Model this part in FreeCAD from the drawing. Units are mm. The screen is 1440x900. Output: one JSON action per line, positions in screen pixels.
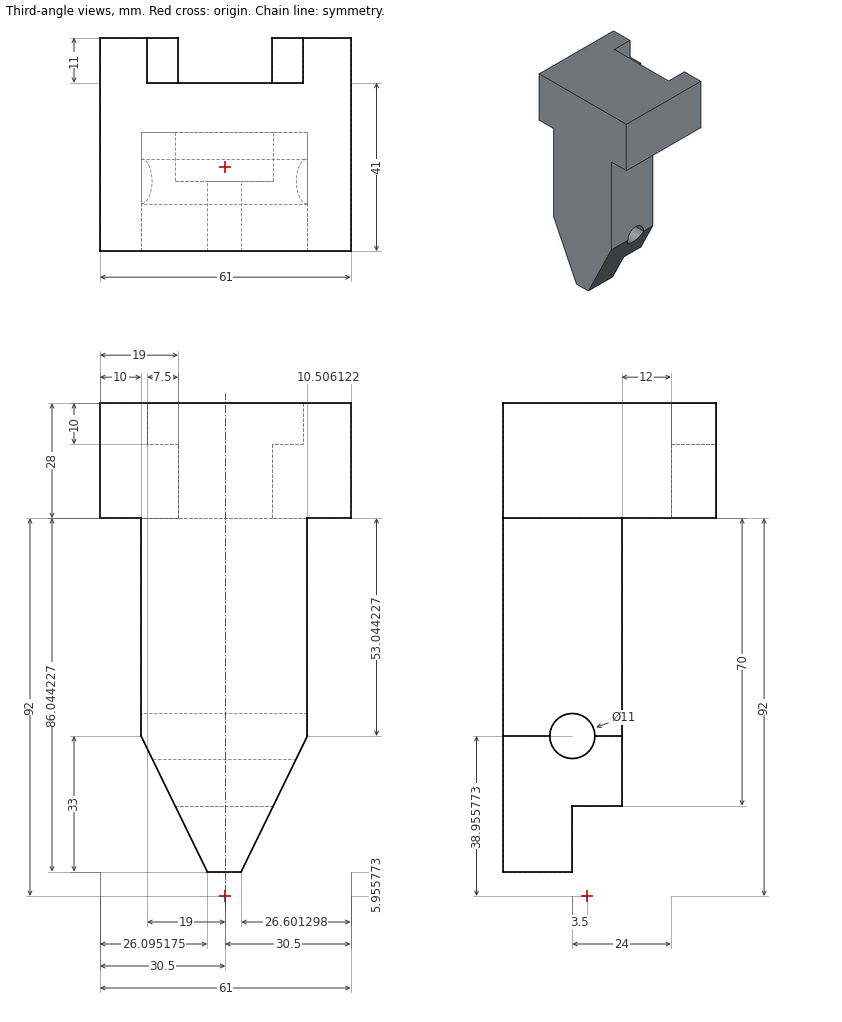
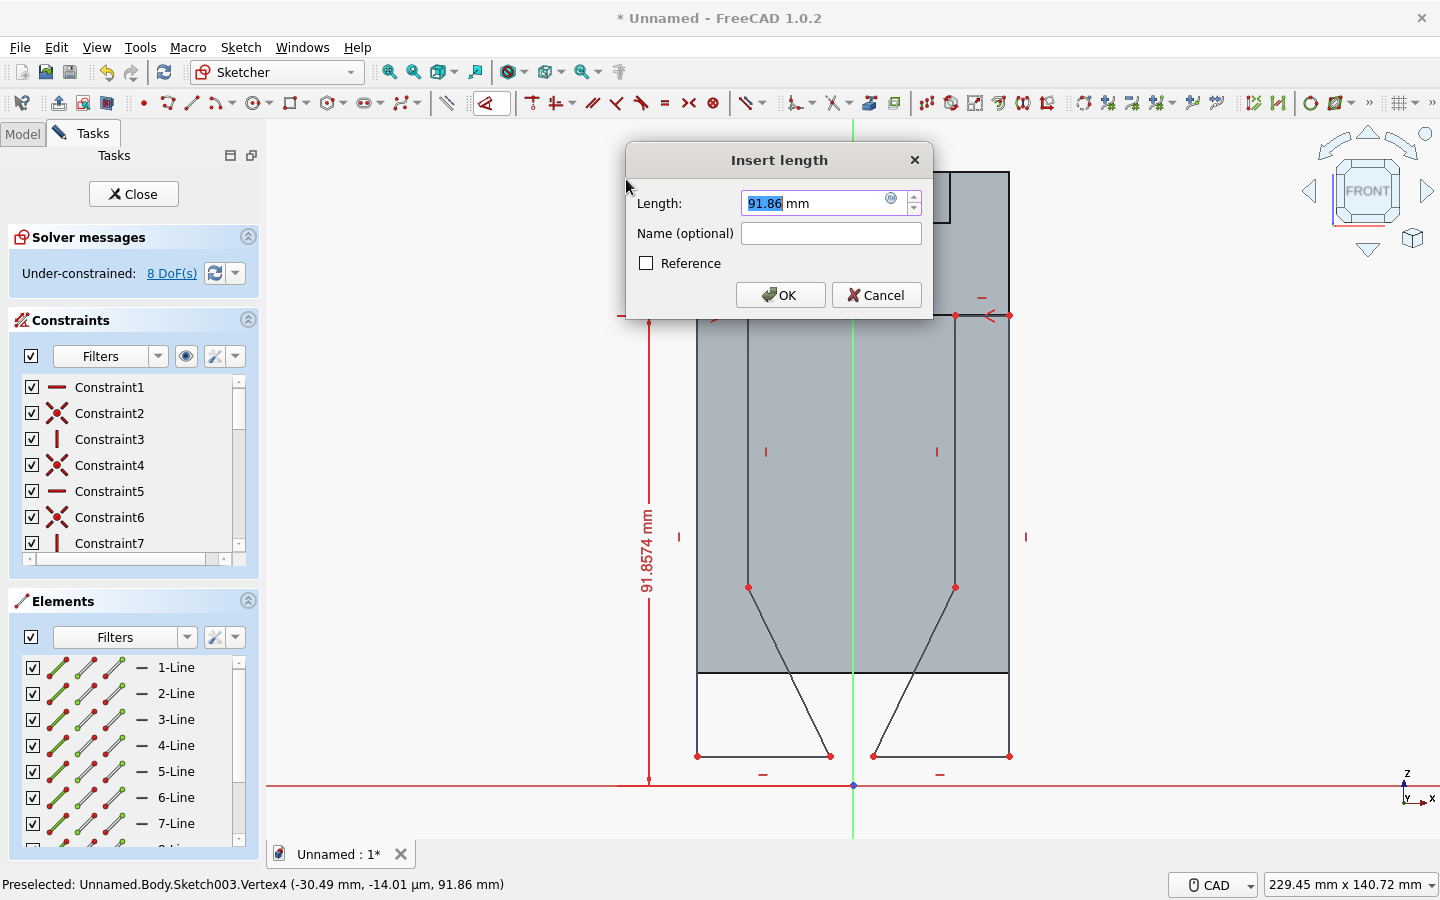
{"action": "type", "text": "92"}
{"action": "key", "text": "Return"}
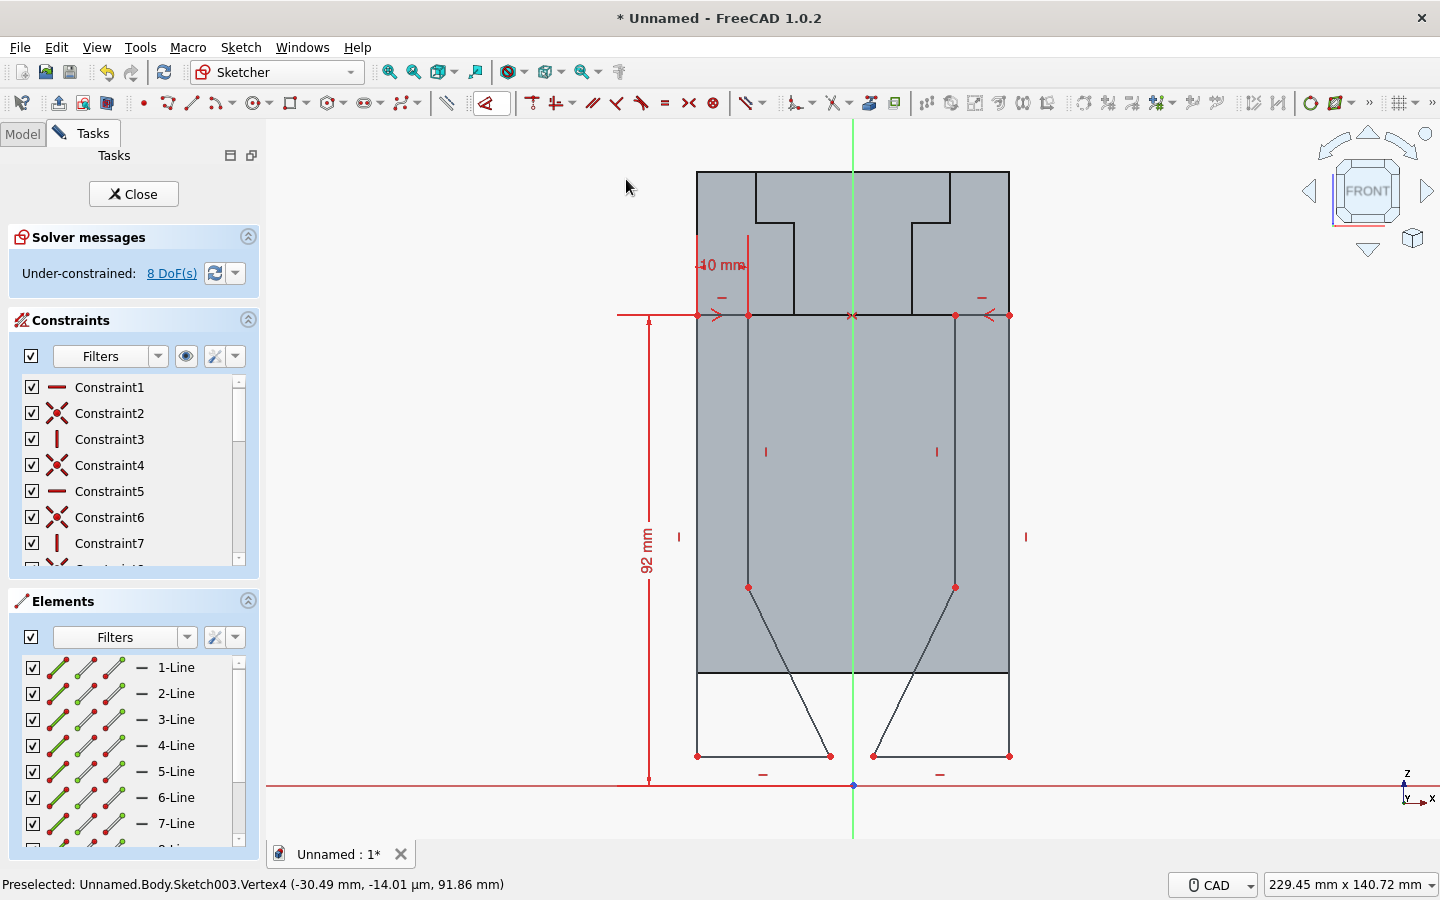
{"action": "left_click", "coordinate": [773, 639]}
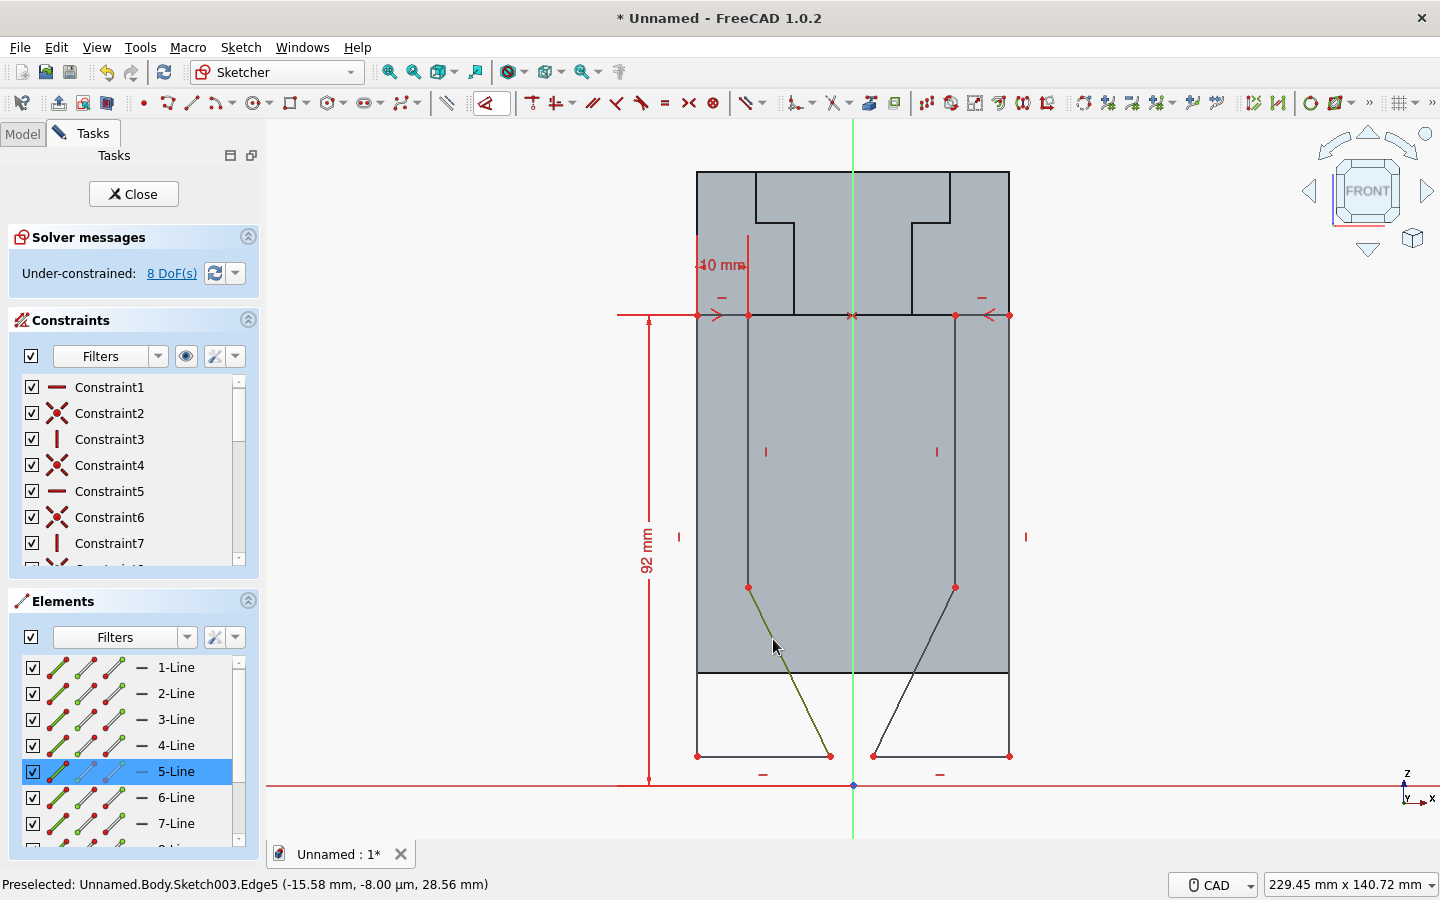
{"action": "left_click", "coordinate": [504, 104]}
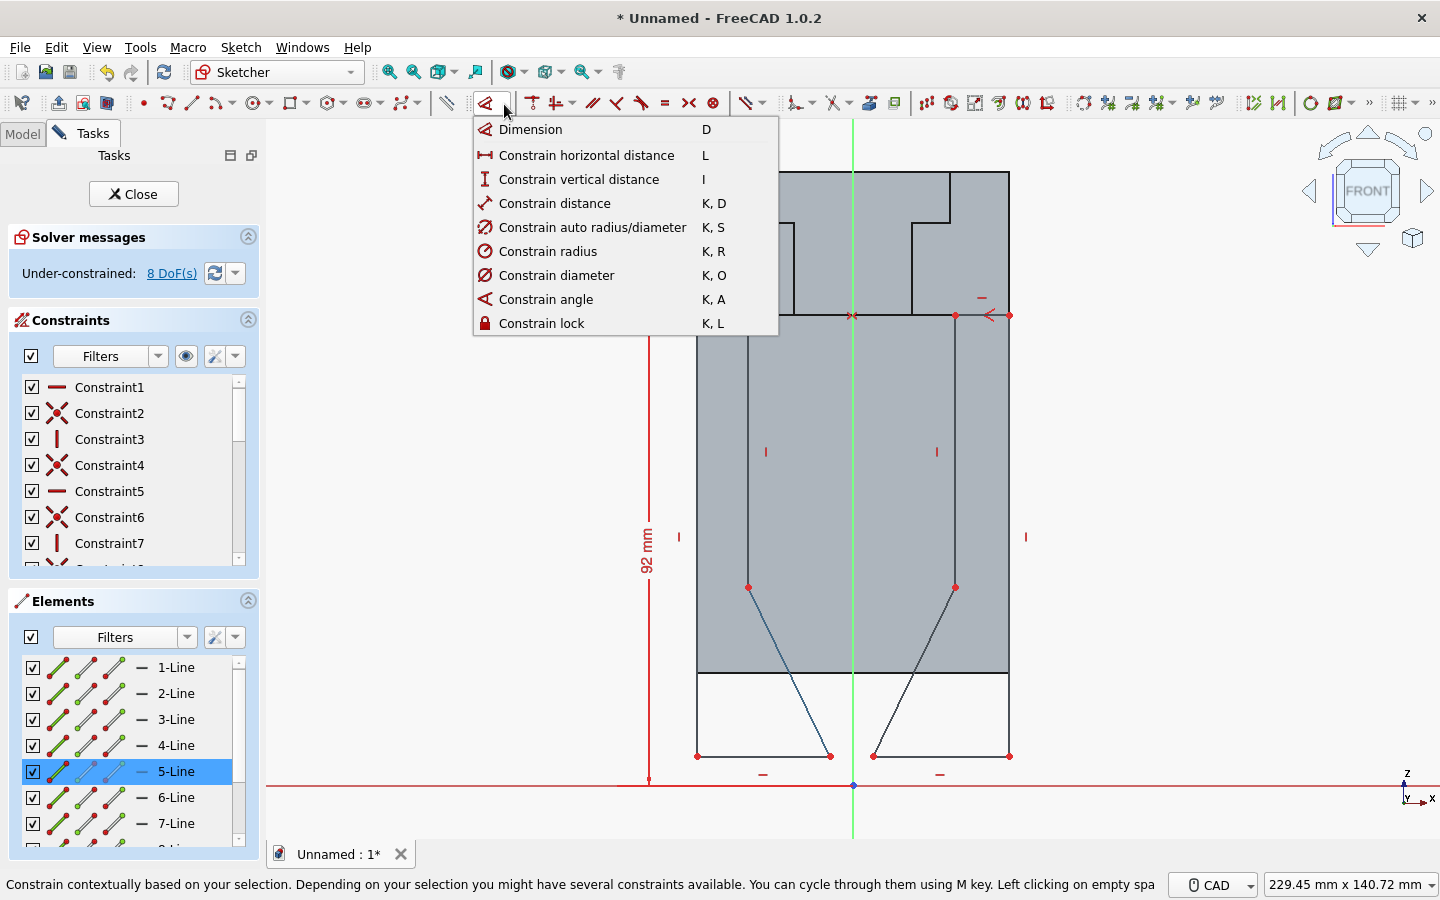
{"action": "left_click", "coordinate": [626, 179]}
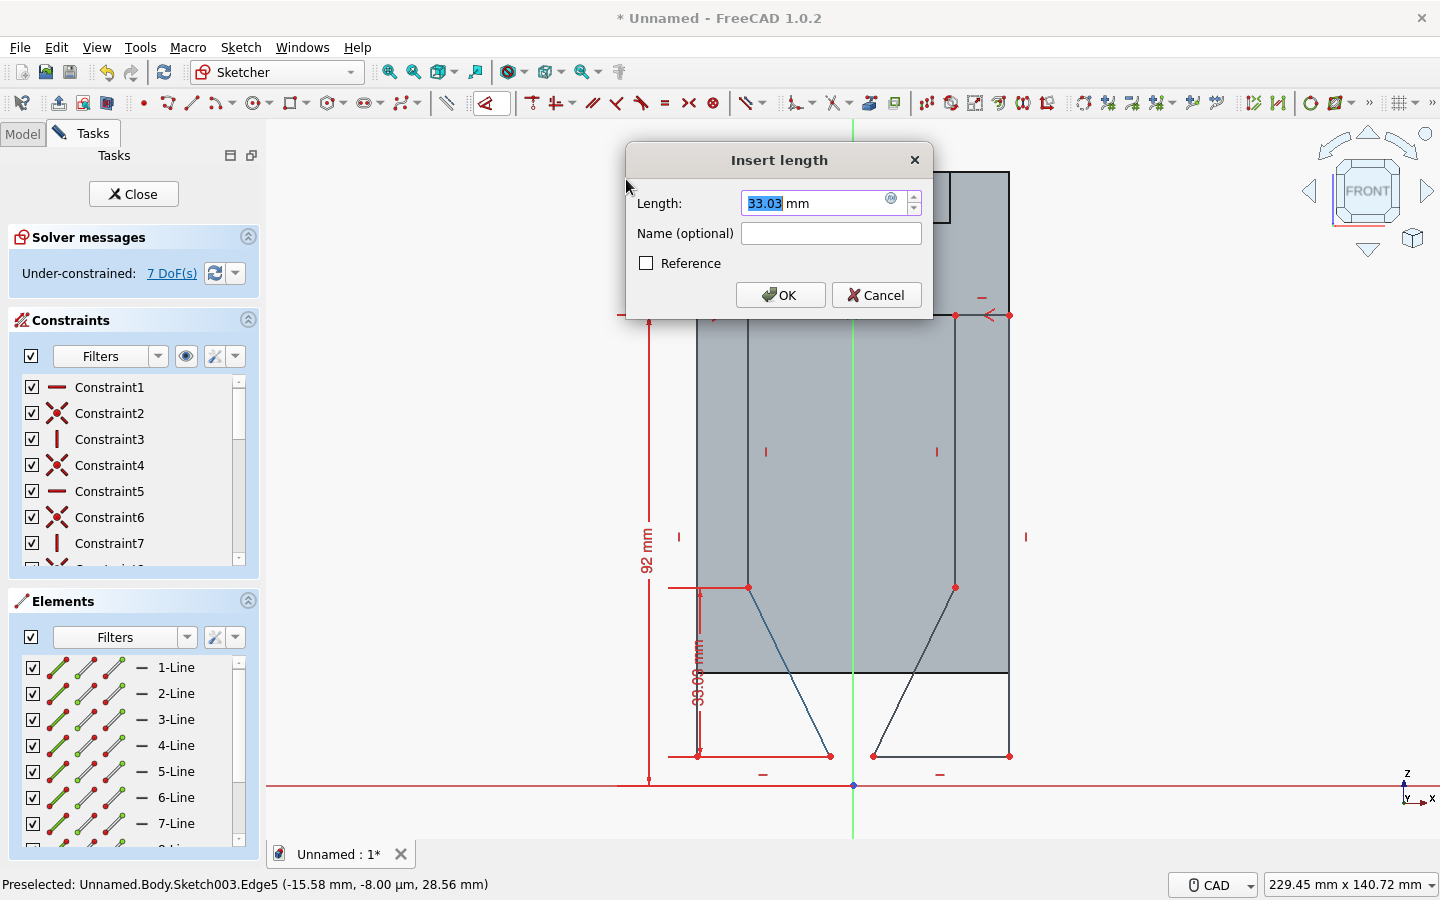
{"action": "type", "text": "33"}
{"action": "key", "text": "Return"}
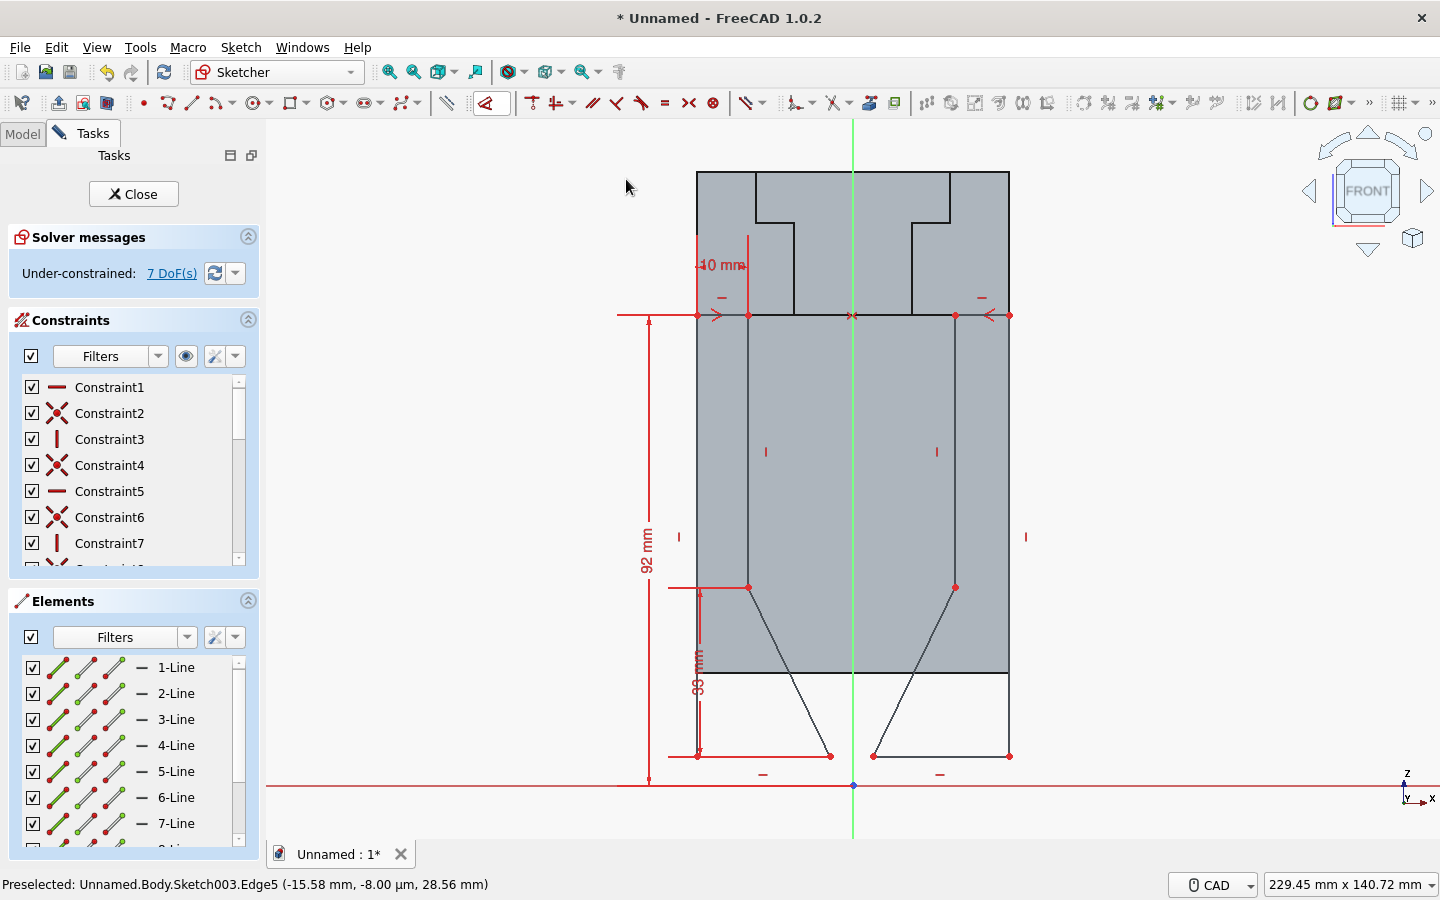
{"action": "left_click", "coordinate": [898, 706]}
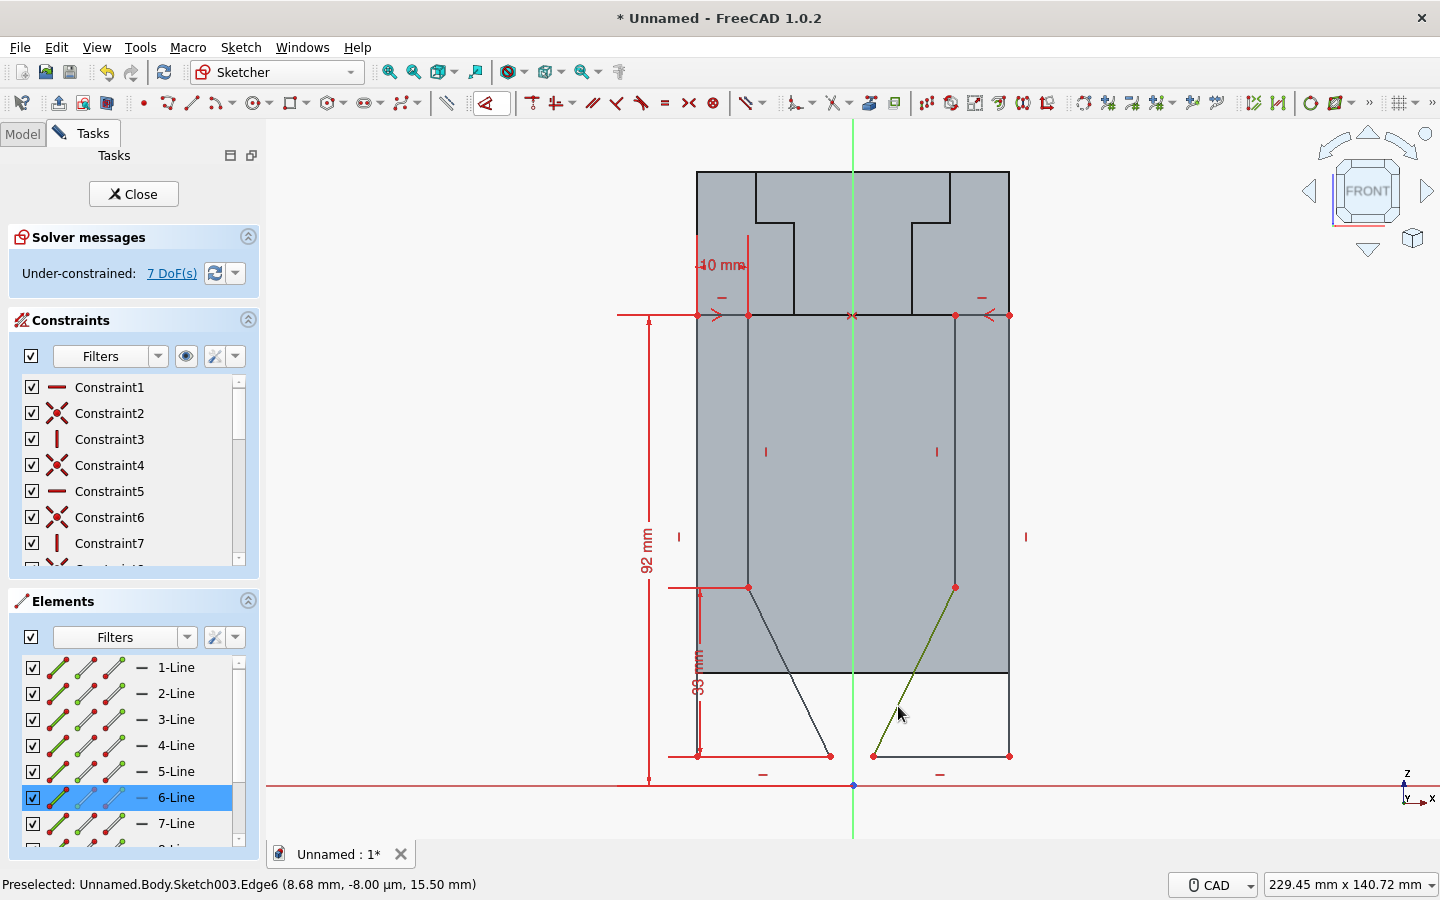
{"action": "left_click", "coordinate": [504, 104]}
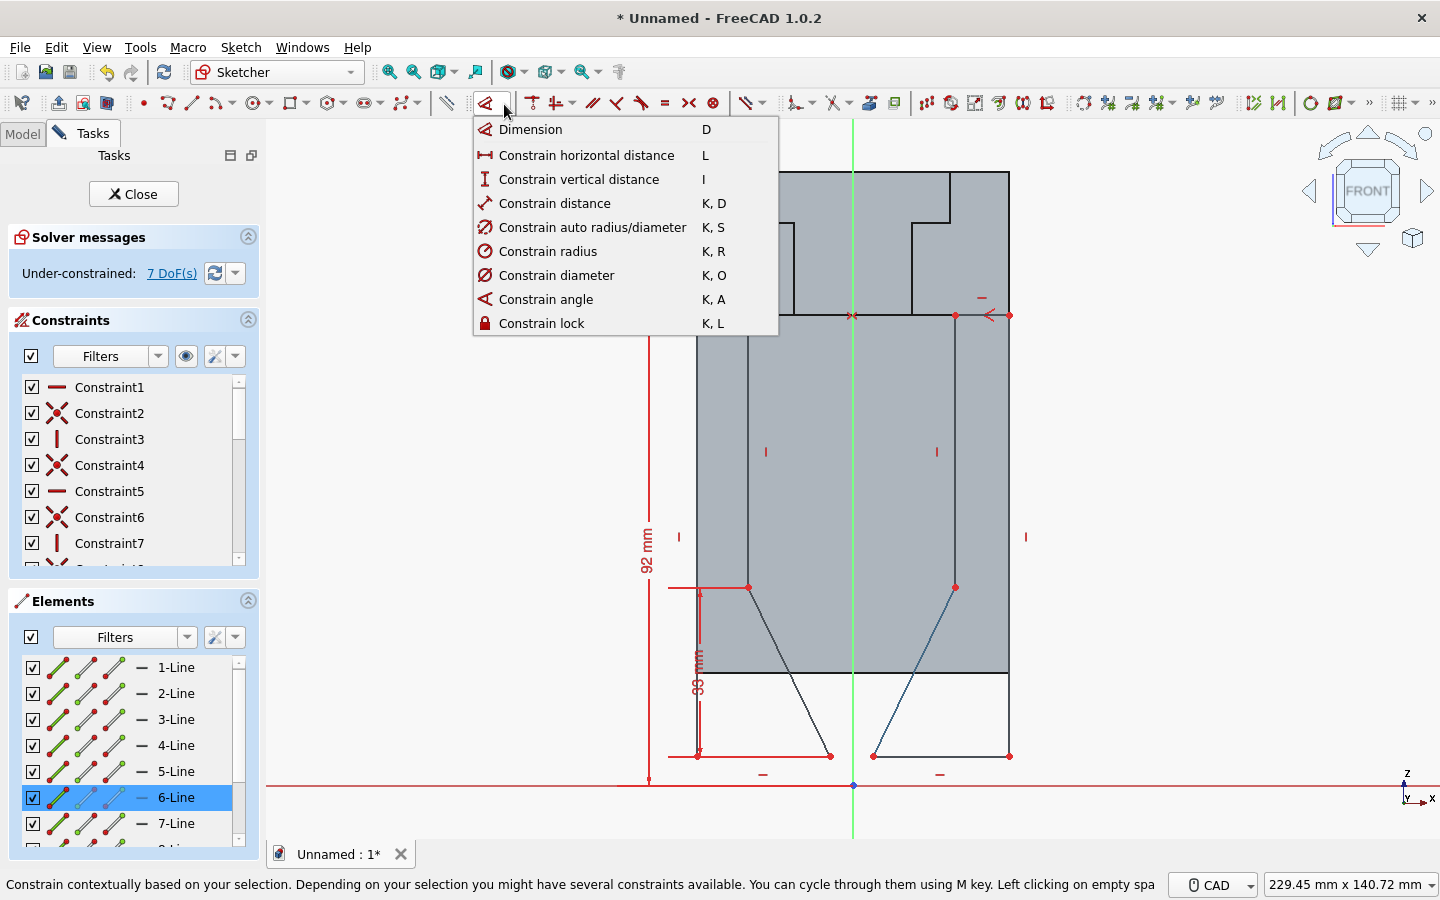
{"action": "left_click", "coordinate": [626, 179]}